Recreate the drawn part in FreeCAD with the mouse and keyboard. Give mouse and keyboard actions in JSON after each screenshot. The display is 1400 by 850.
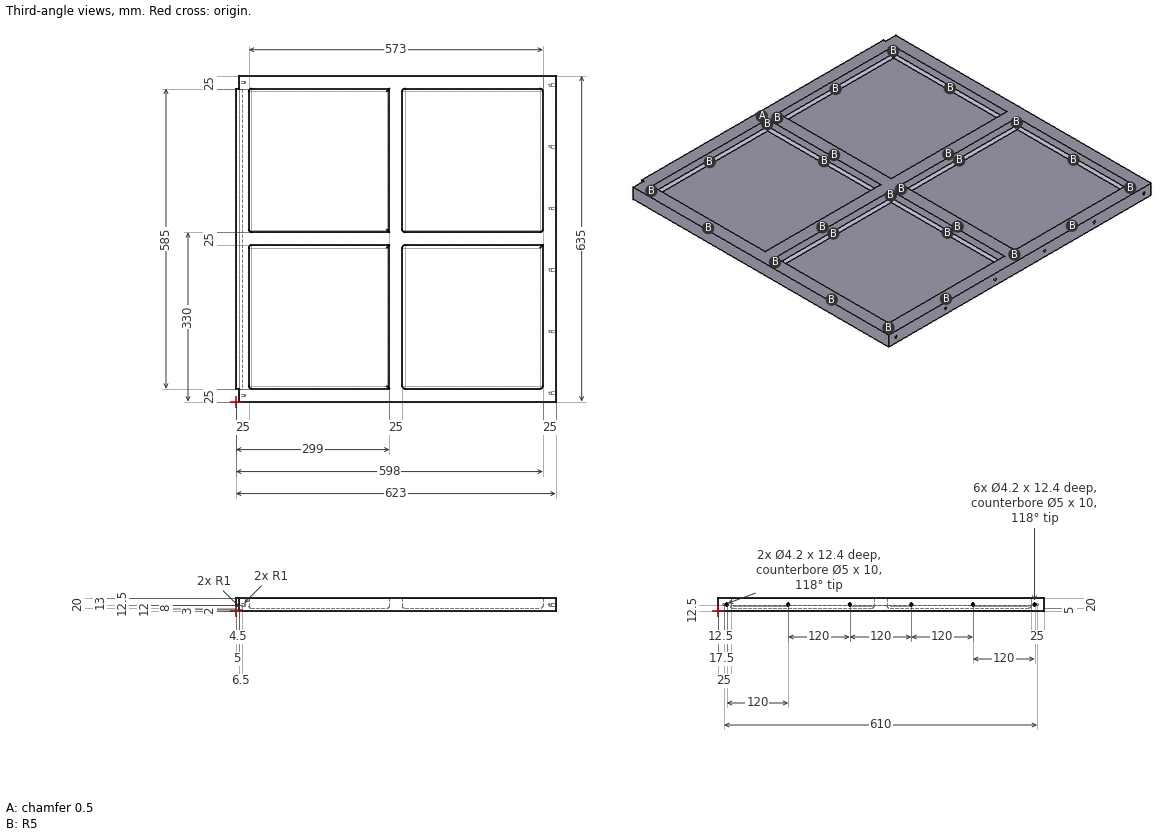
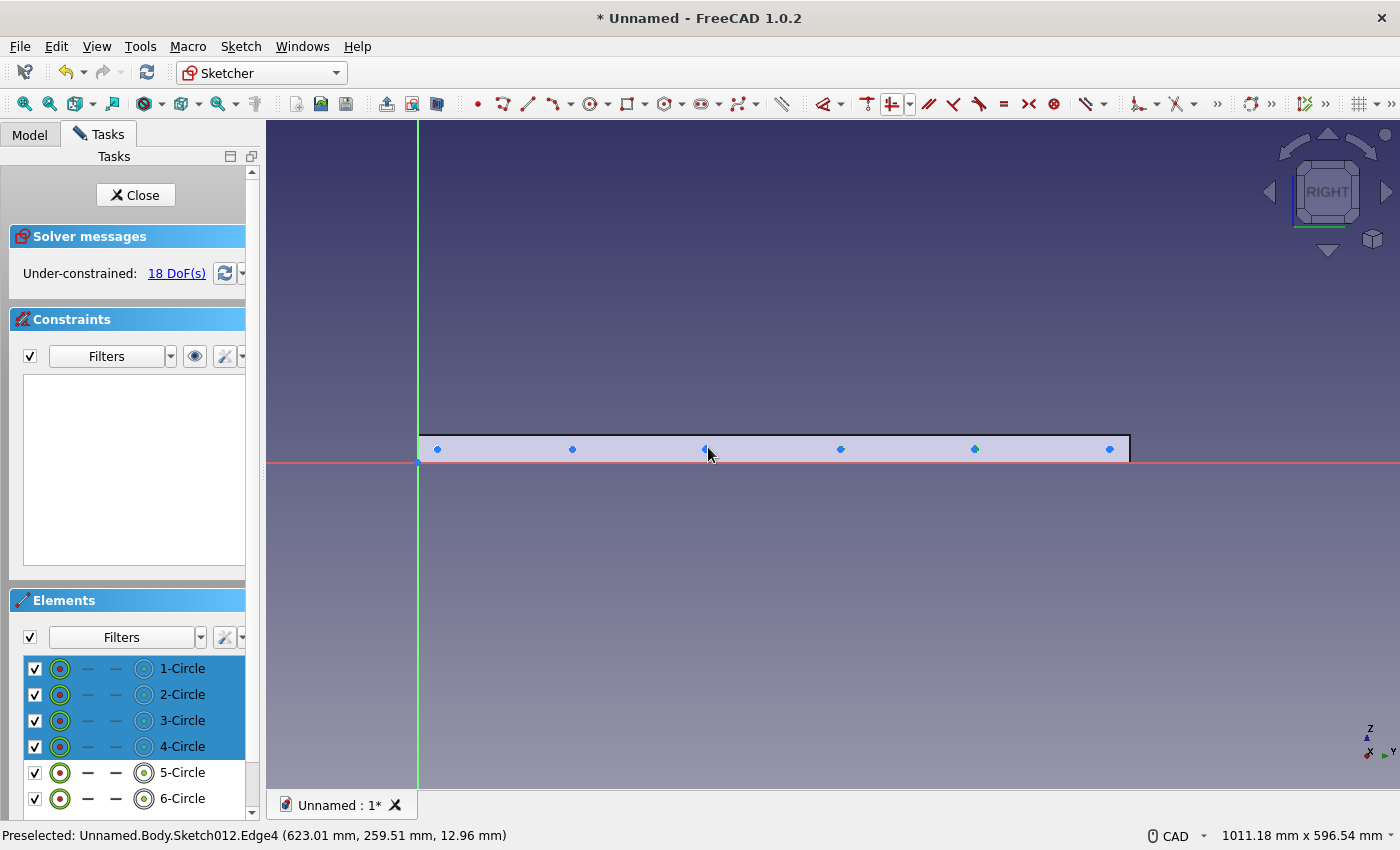
{"action": "scroll", "coordinate": [574, 447], "scroll_direction": "up", "scroll_amount": 9}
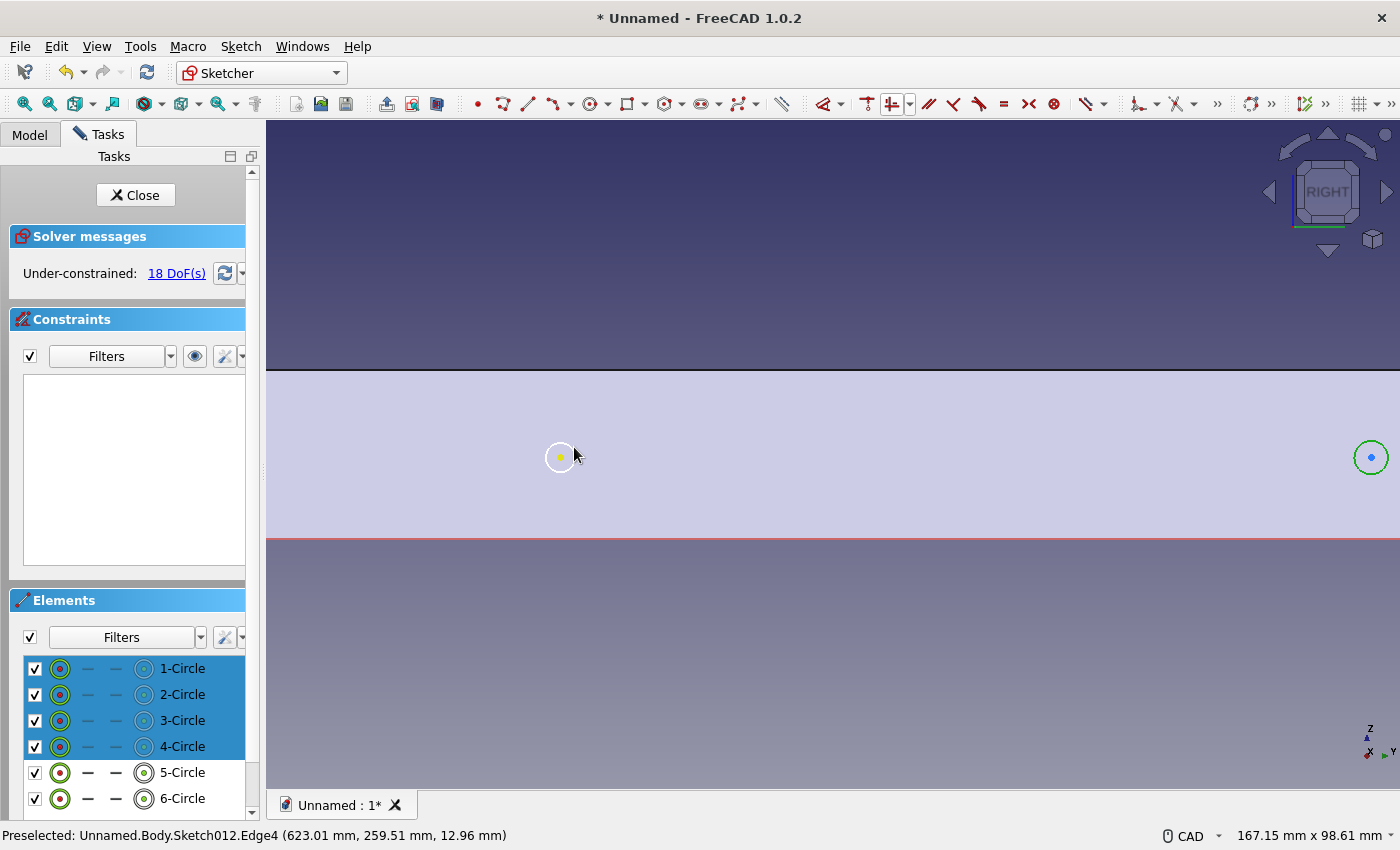
{"action": "left_click", "coordinate": [571, 447]}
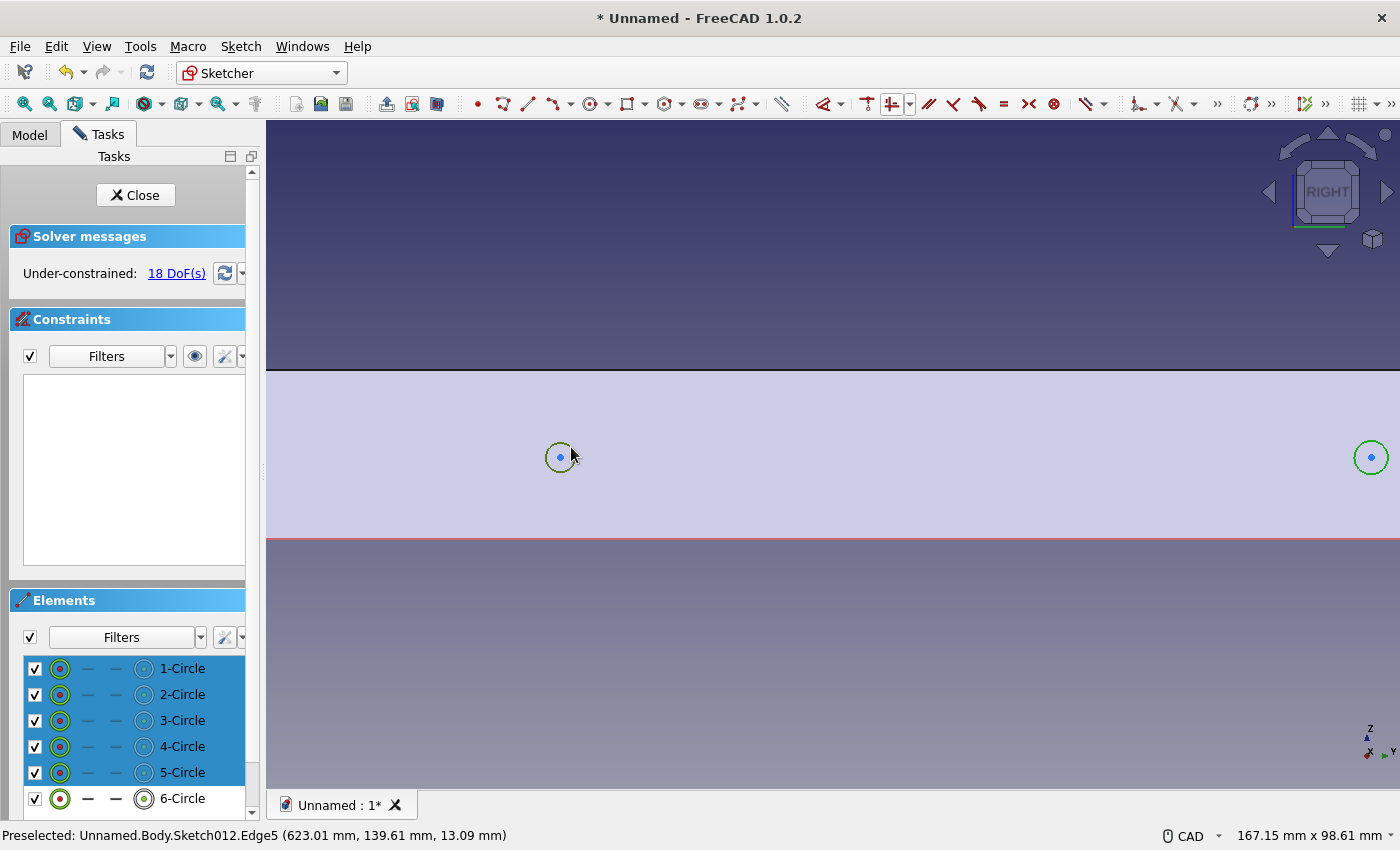
{"action": "scroll", "coordinate": [574, 447], "scroll_direction": "down", "scroll_amount": 9}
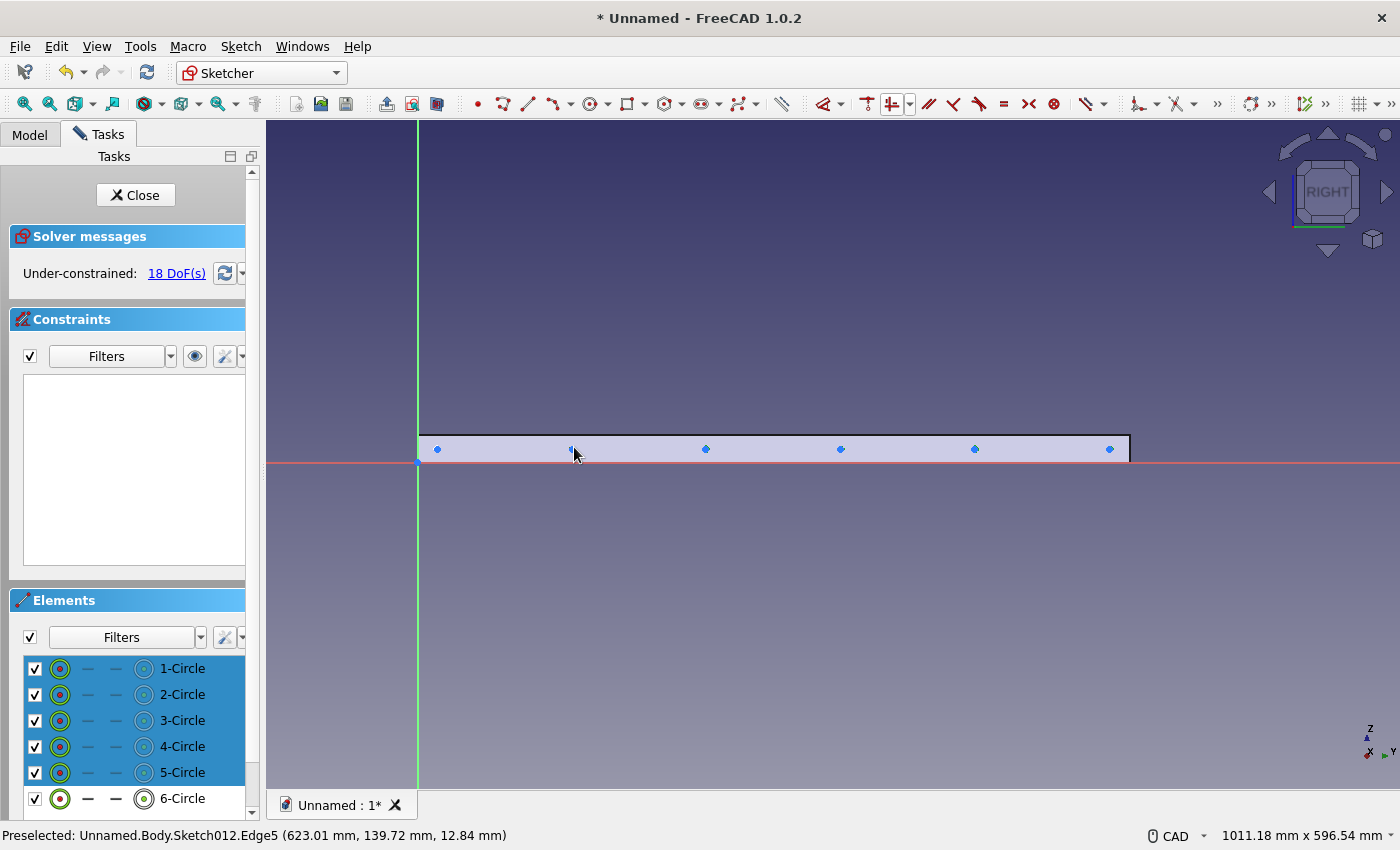
{"action": "scroll", "coordinate": [439, 447], "scroll_direction": "up", "scroll_amount": 9}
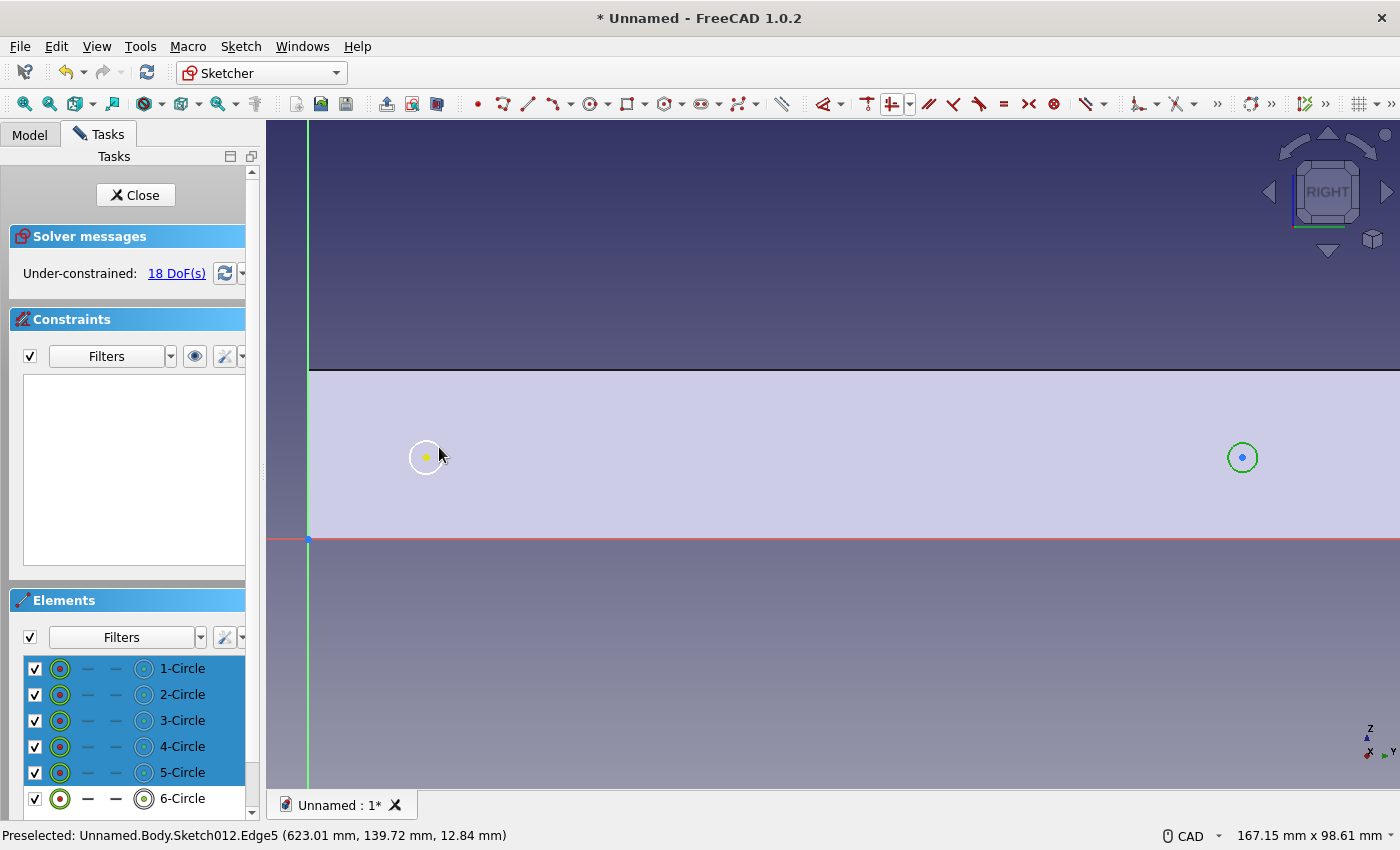
{"action": "left_click", "coordinate": [438, 446]}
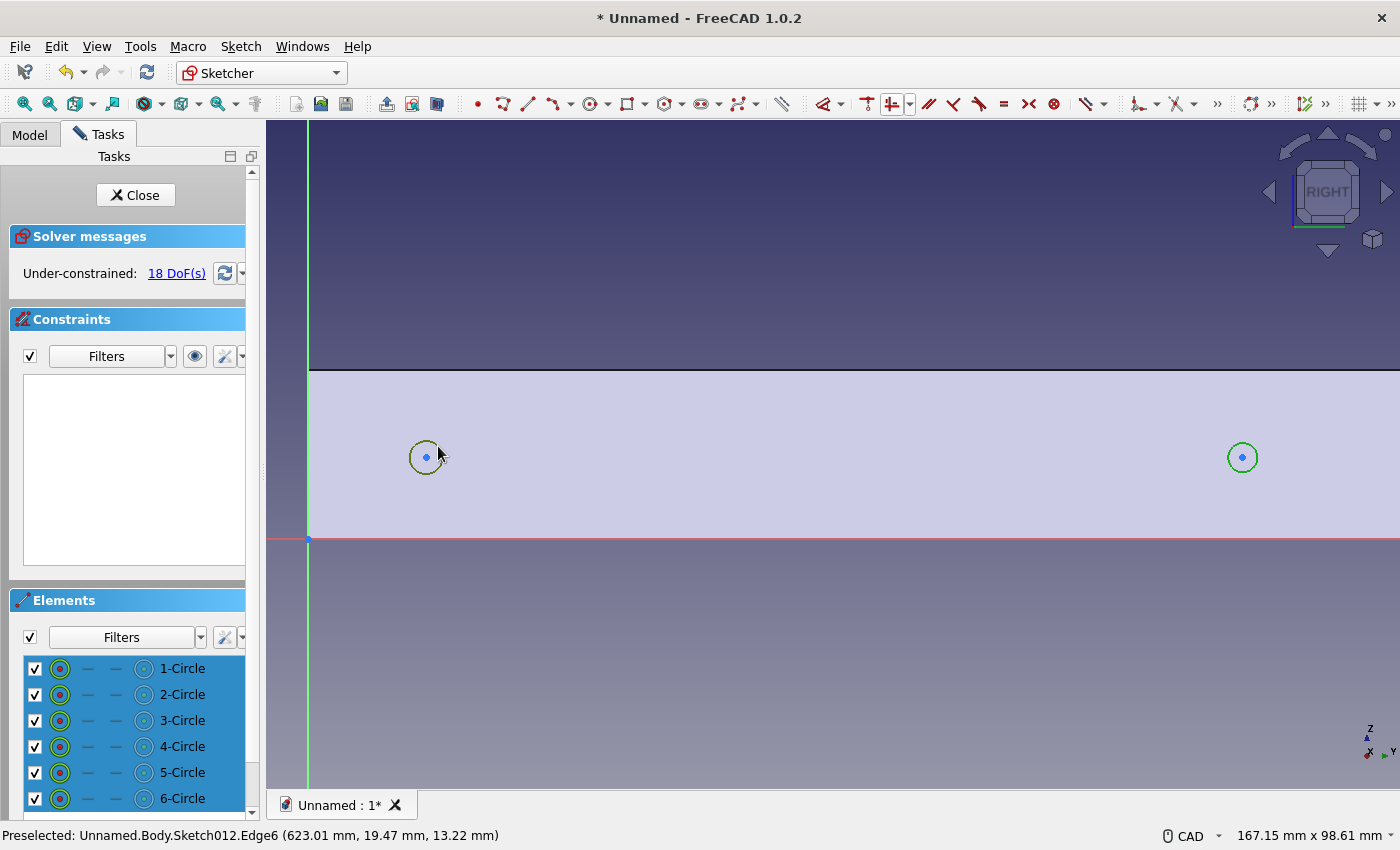
{"action": "left_click", "coordinate": [1004, 104]}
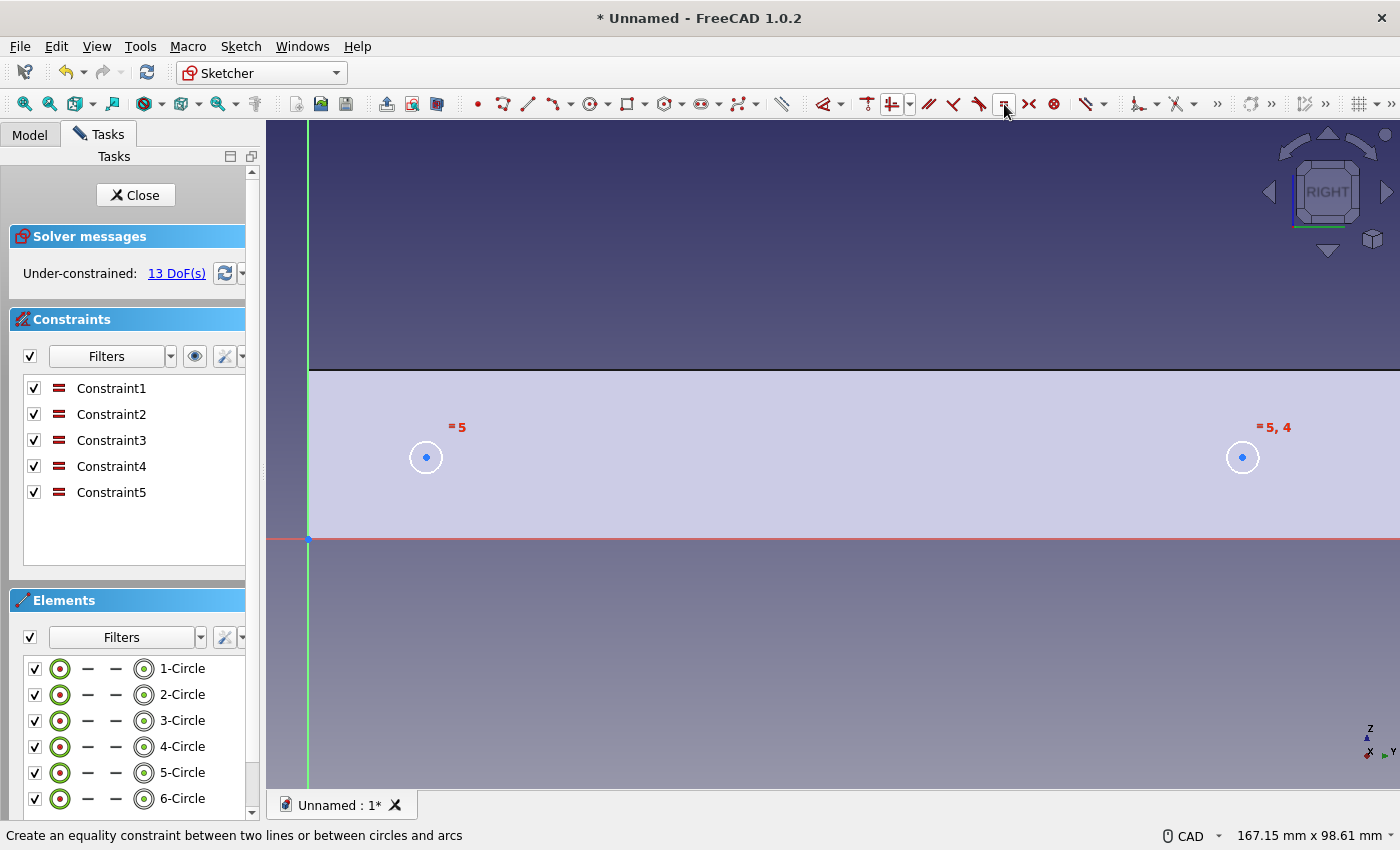
{"action": "left_click", "coordinate": [822, 104]}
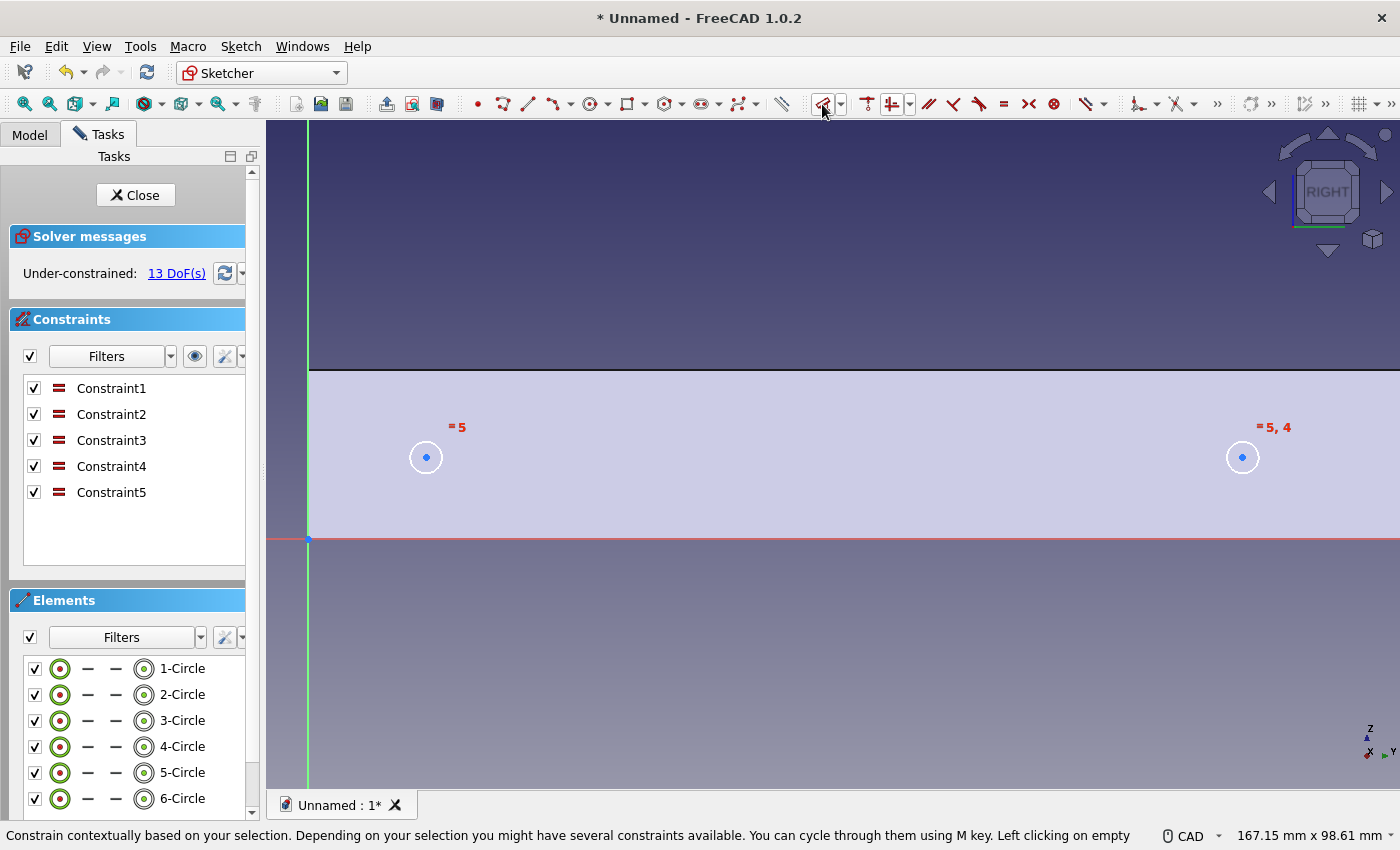
{"action": "scroll", "coordinate": [439, 447], "scroll_direction": "down", "scroll_amount": 9}